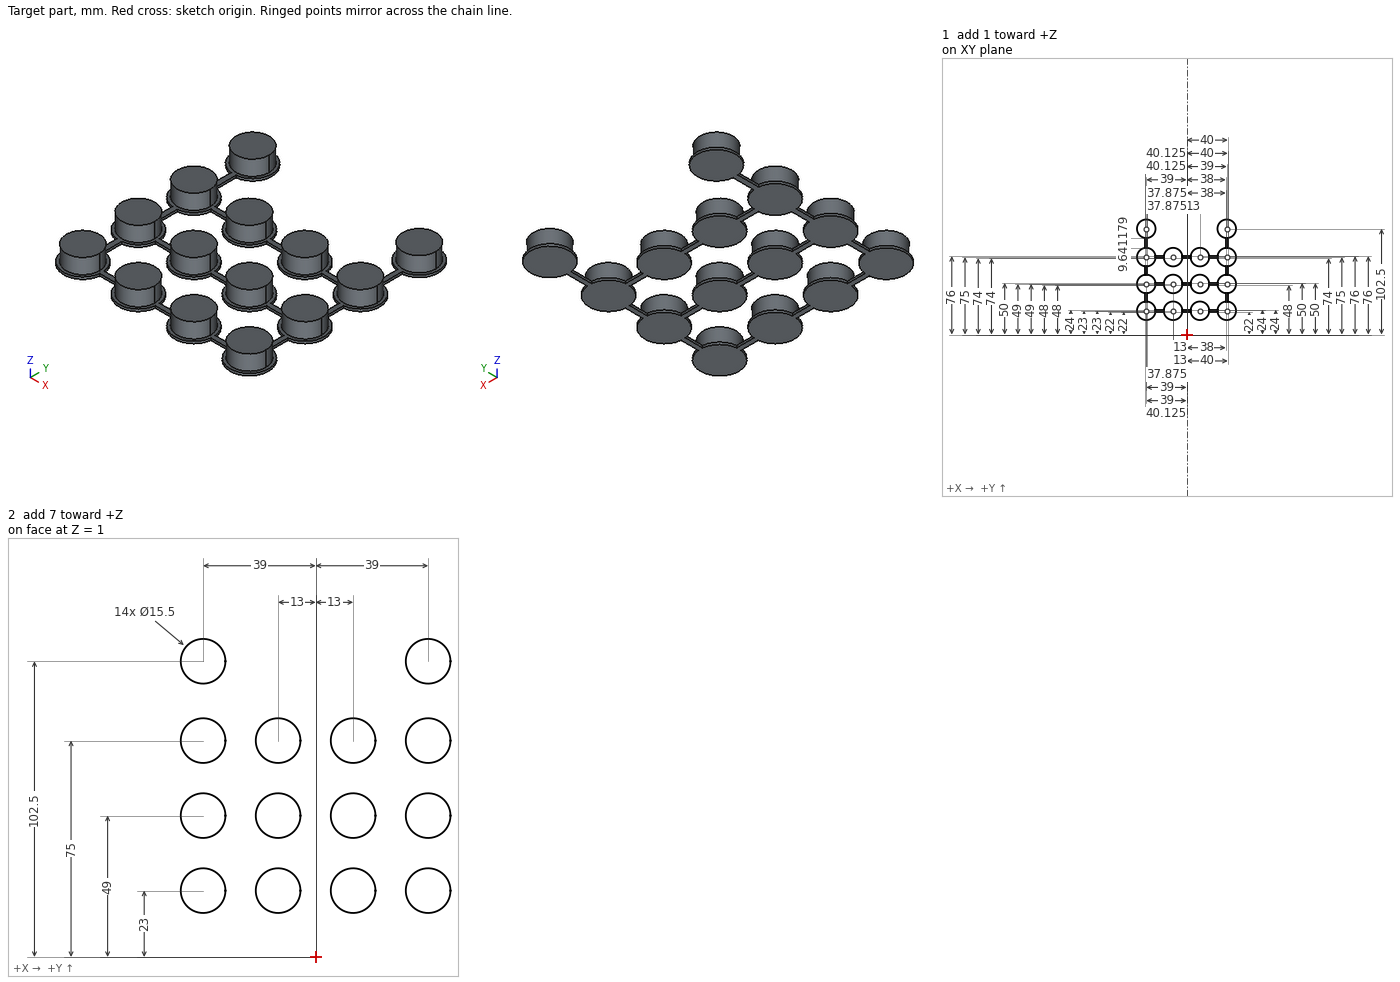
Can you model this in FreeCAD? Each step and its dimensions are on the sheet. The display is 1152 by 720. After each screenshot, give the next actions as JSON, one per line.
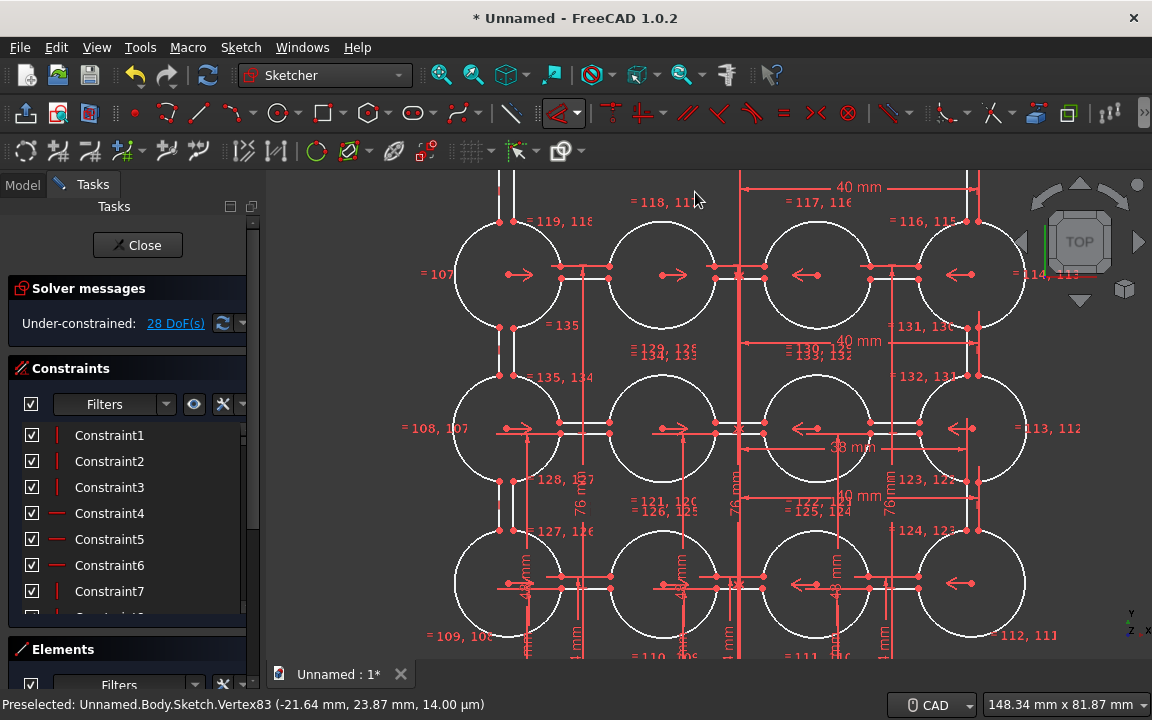
{"action": "left_click", "coordinate": [562, 279]}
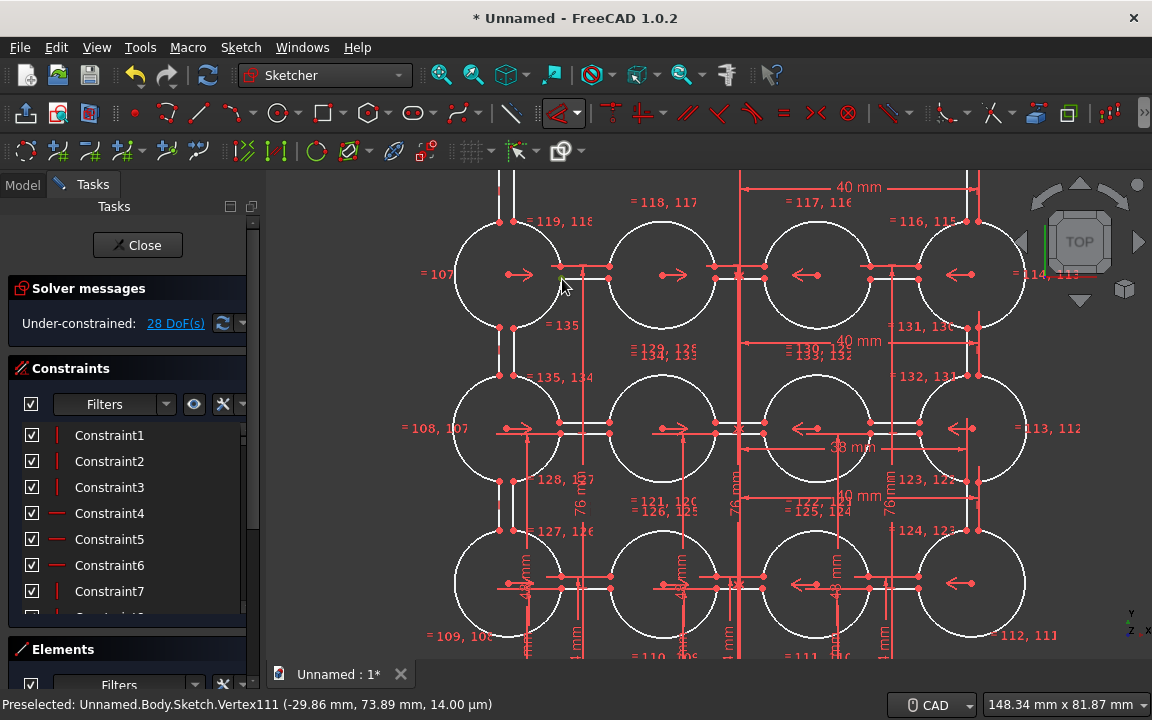
{"action": "left_click", "coordinate": [580, 114]}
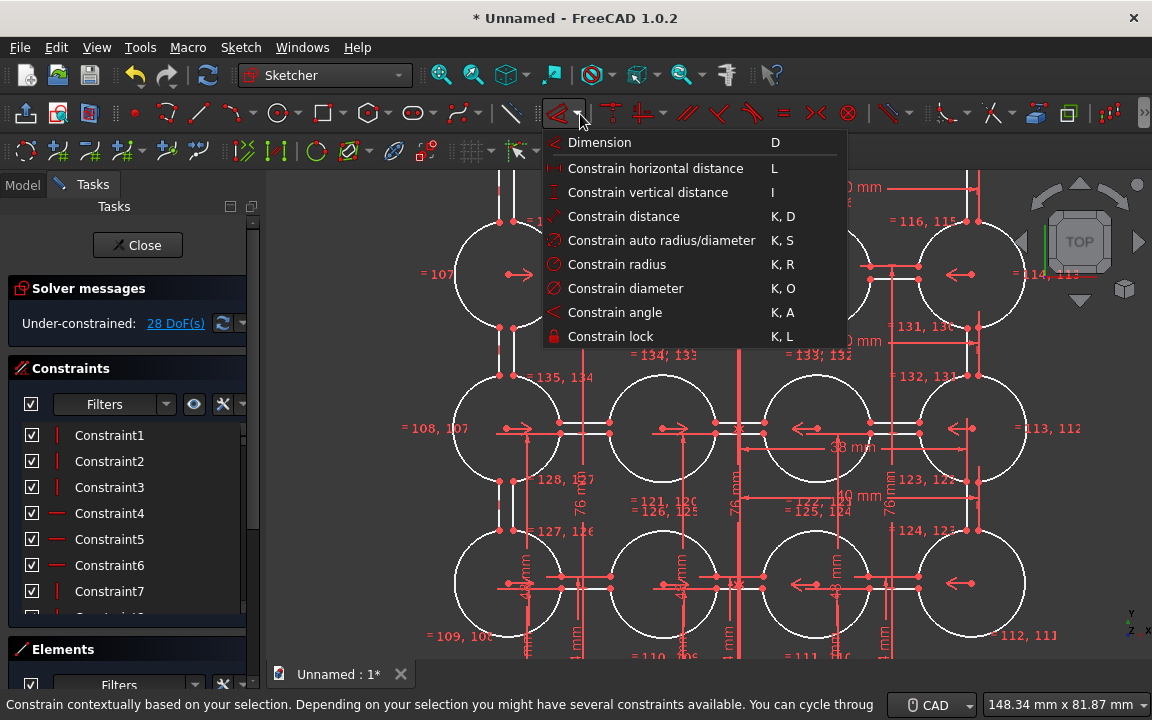
{"action": "left_click", "coordinate": [695, 192]}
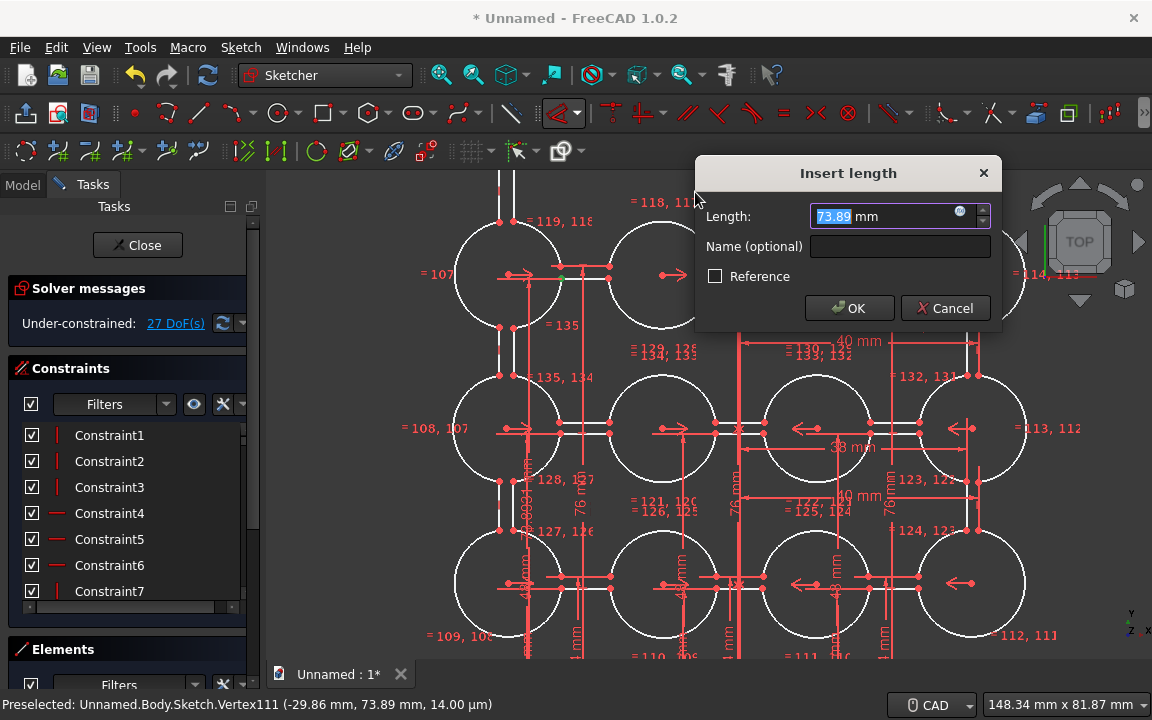
{"action": "type", "text": "74"}
{"action": "key", "text": "Return"}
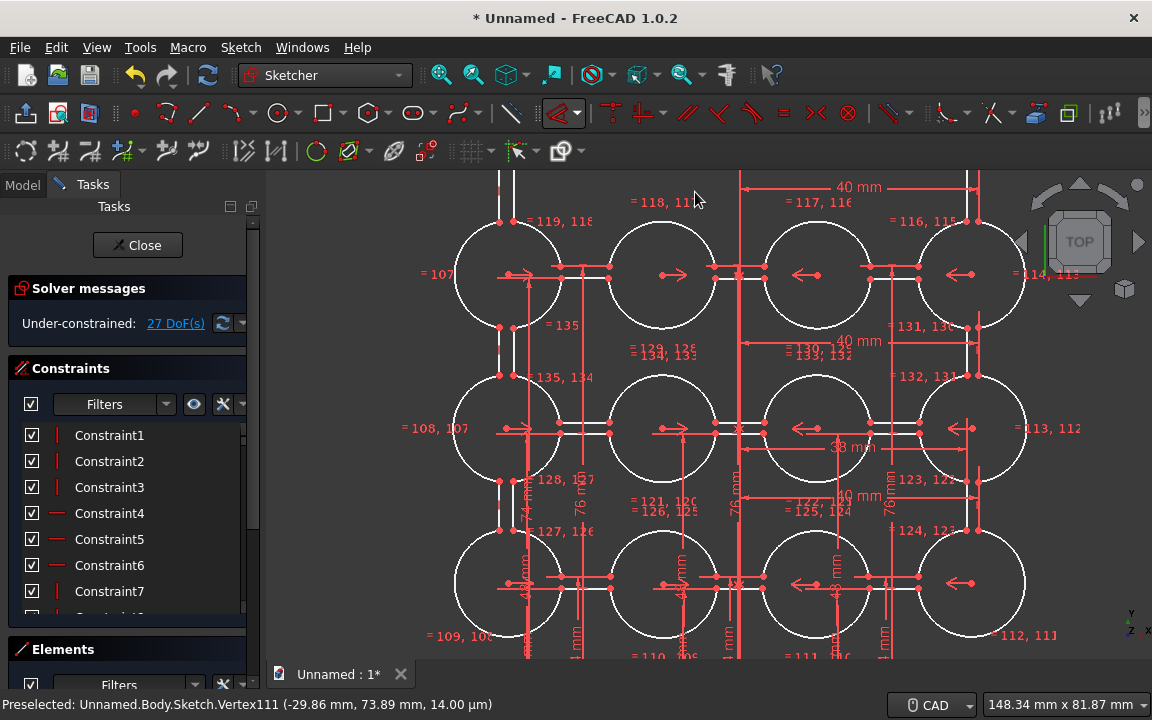
{"action": "left_click", "coordinate": [715, 279]}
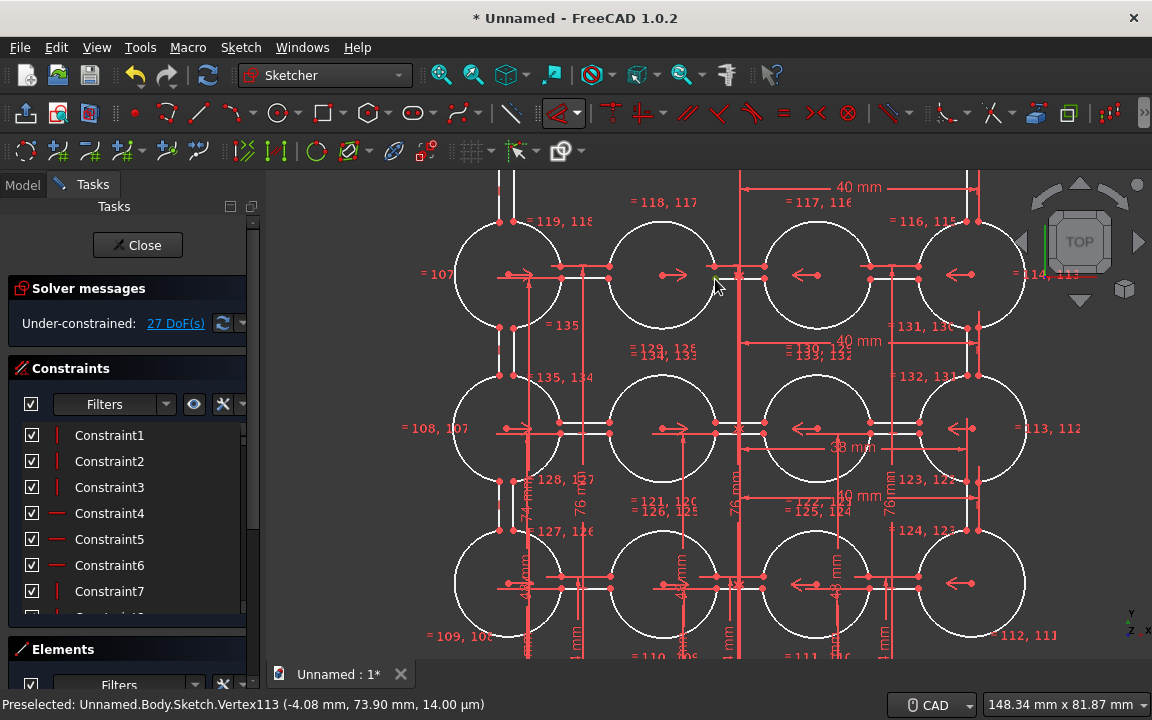
{"action": "key", "text": "i"}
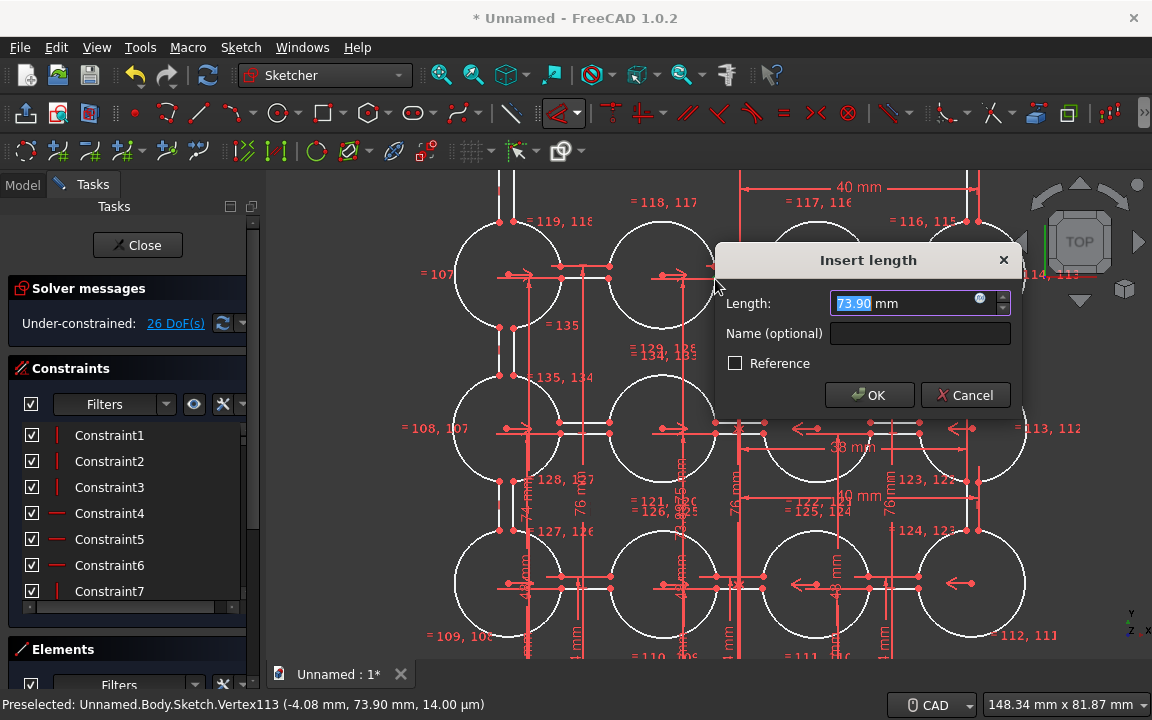
{"action": "type", "text": "74"}
{"action": "key", "text": "Return"}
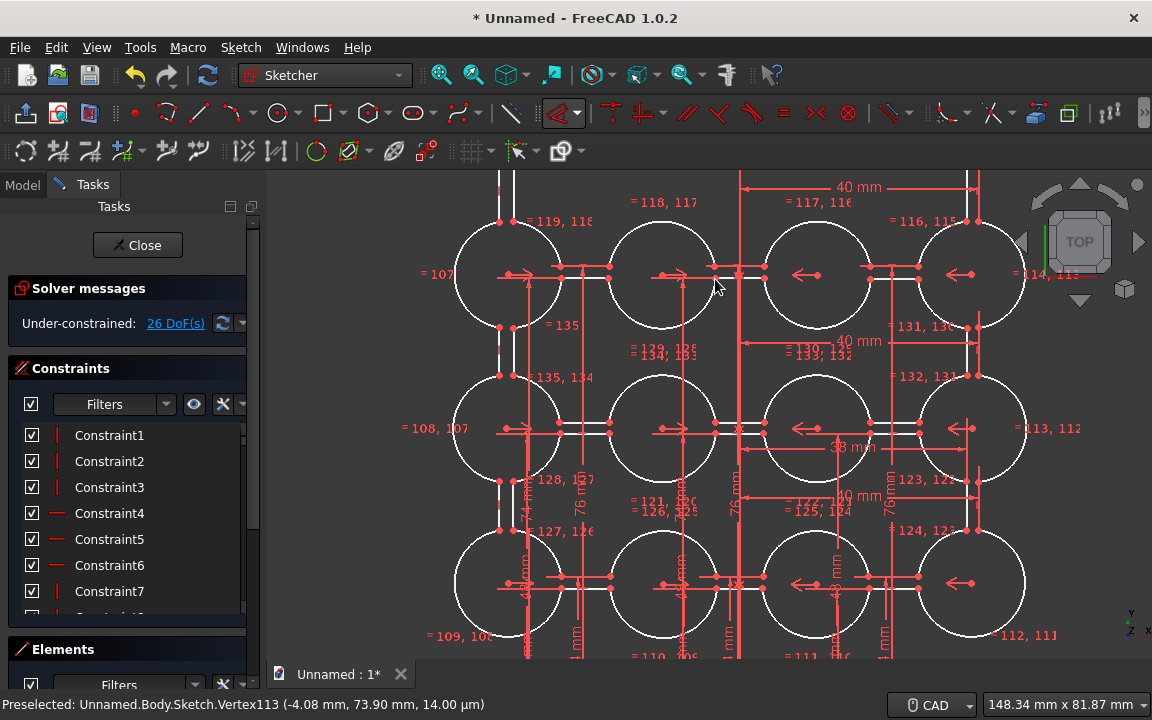
{"action": "left_click", "coordinate": [871, 279]}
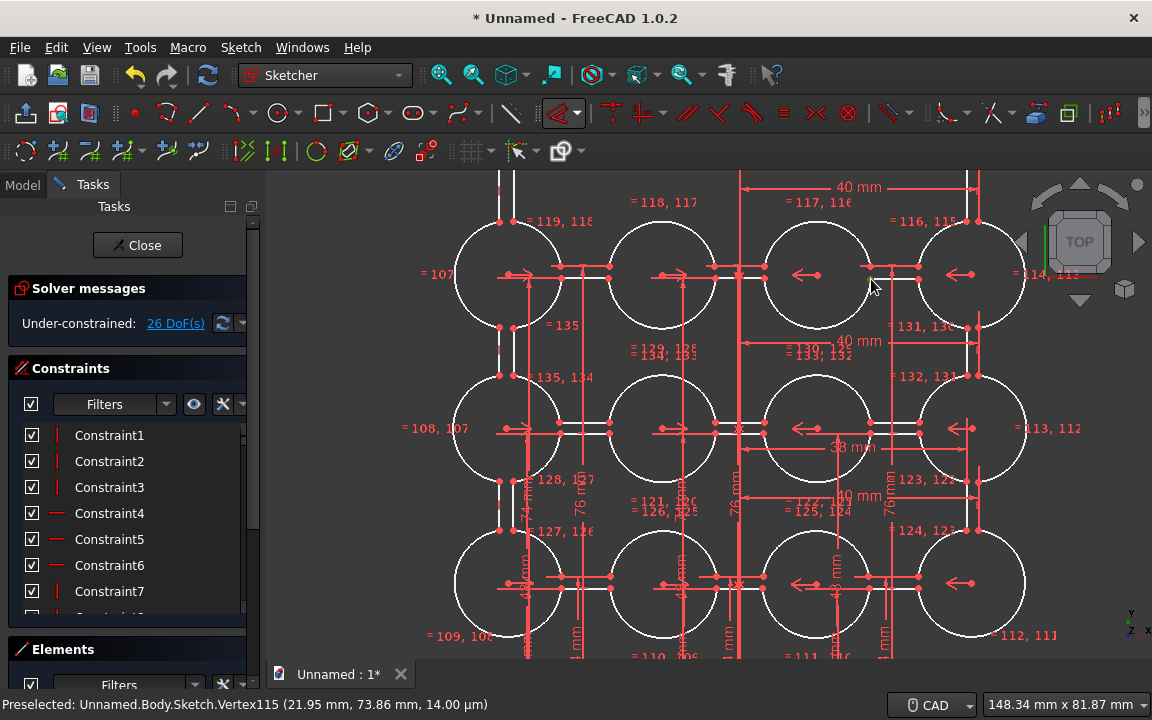
{"action": "left_click", "coordinate": [580, 114]}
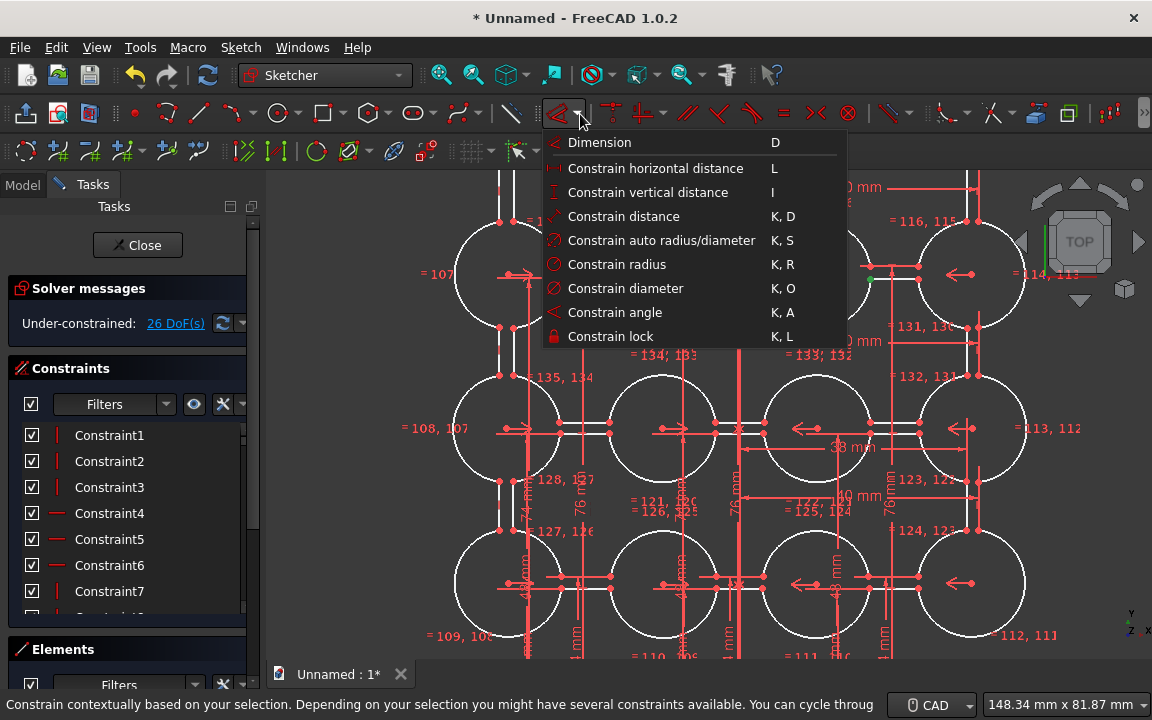
{"action": "left_click", "coordinate": [695, 192]}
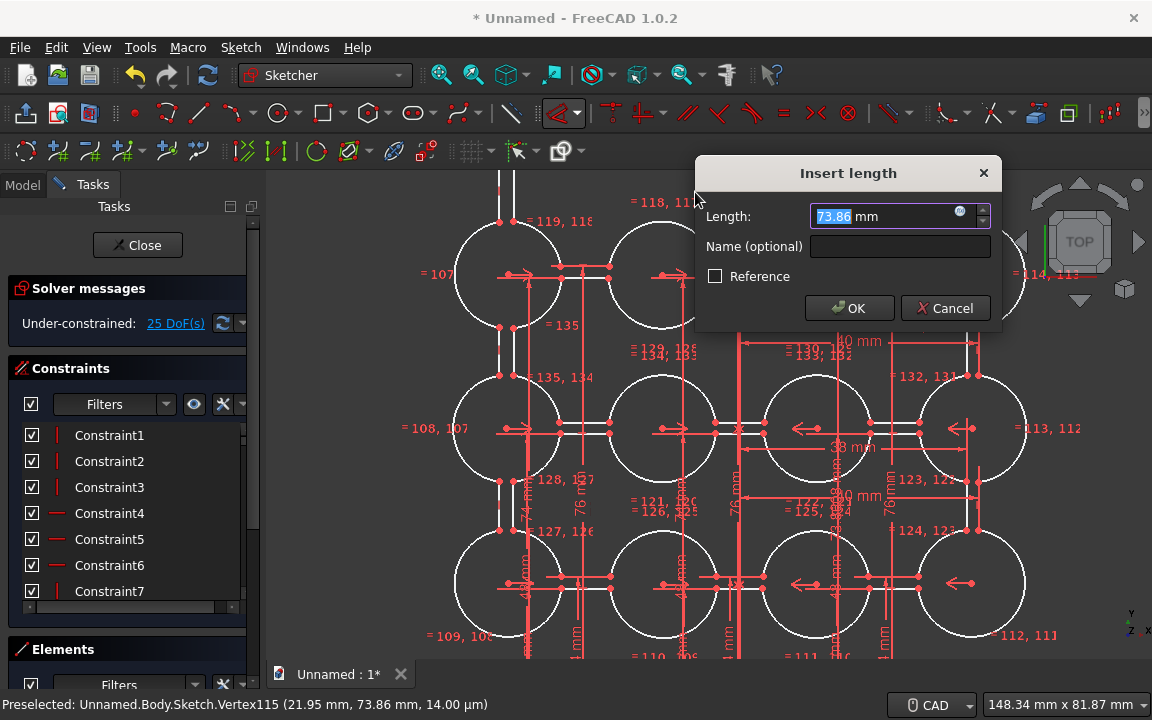
{"action": "type", "text": "74"}
{"action": "key", "text": "Return"}